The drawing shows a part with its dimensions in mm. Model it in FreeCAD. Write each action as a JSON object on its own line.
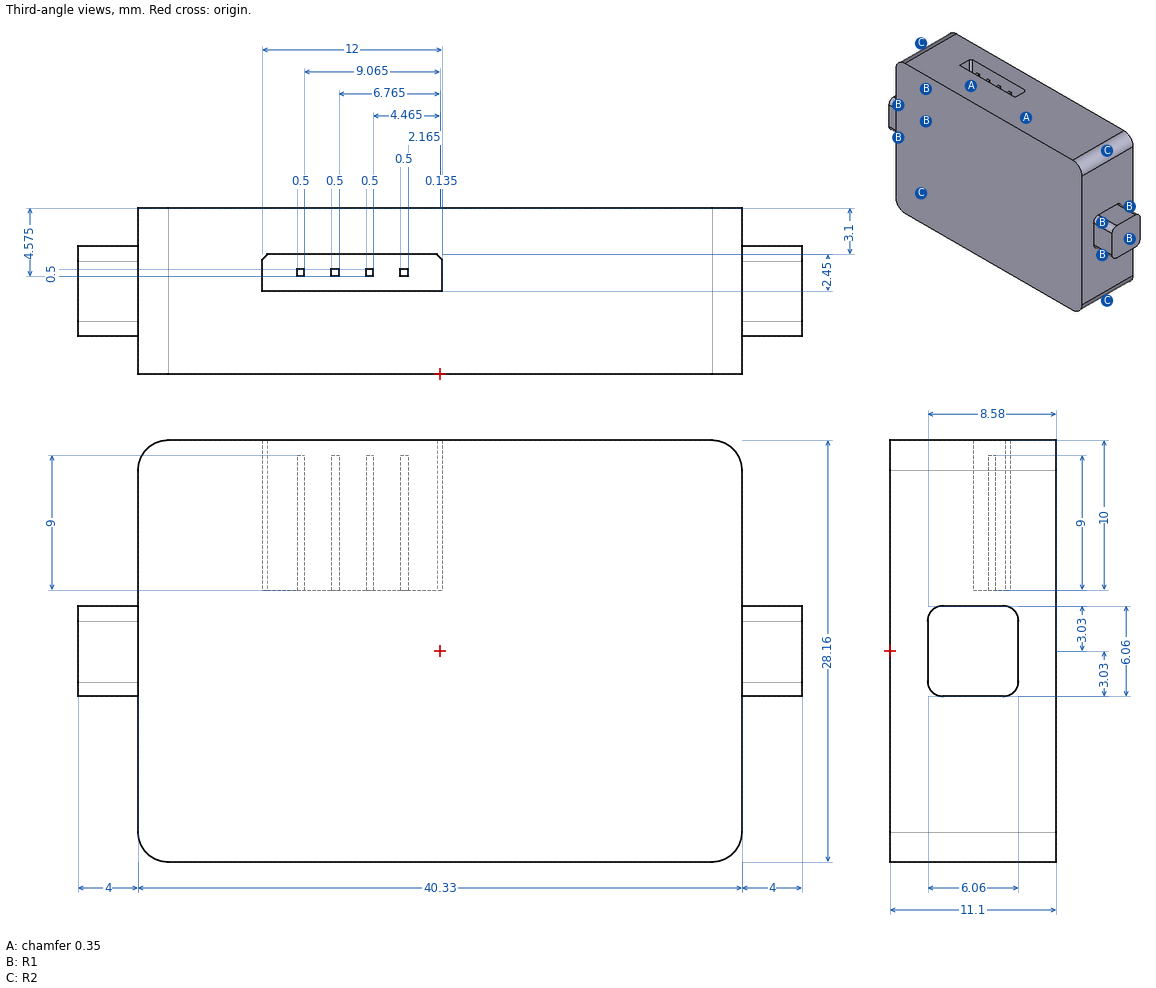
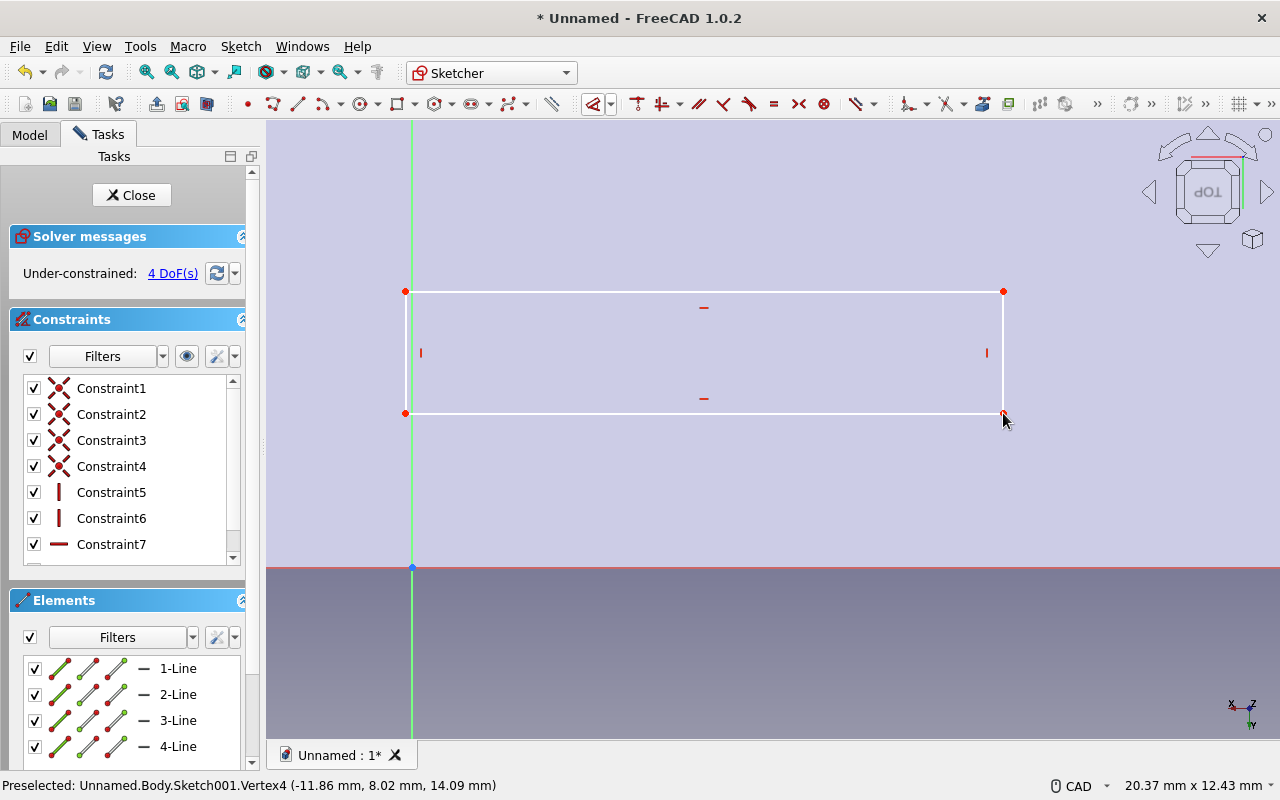
{"action": "key", "text": "d"}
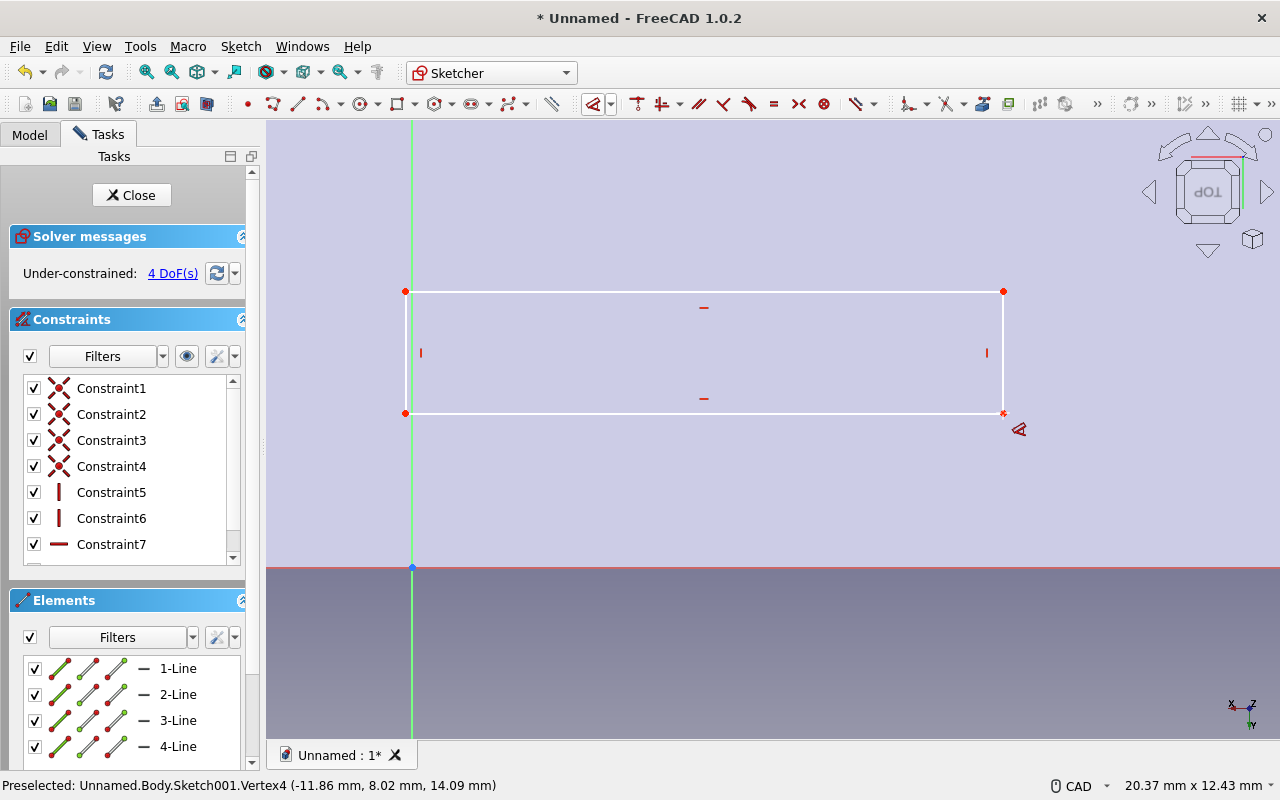
{"action": "left_click", "coordinate": [585, 414]}
{"action": "left_click", "coordinate": [704, 380]}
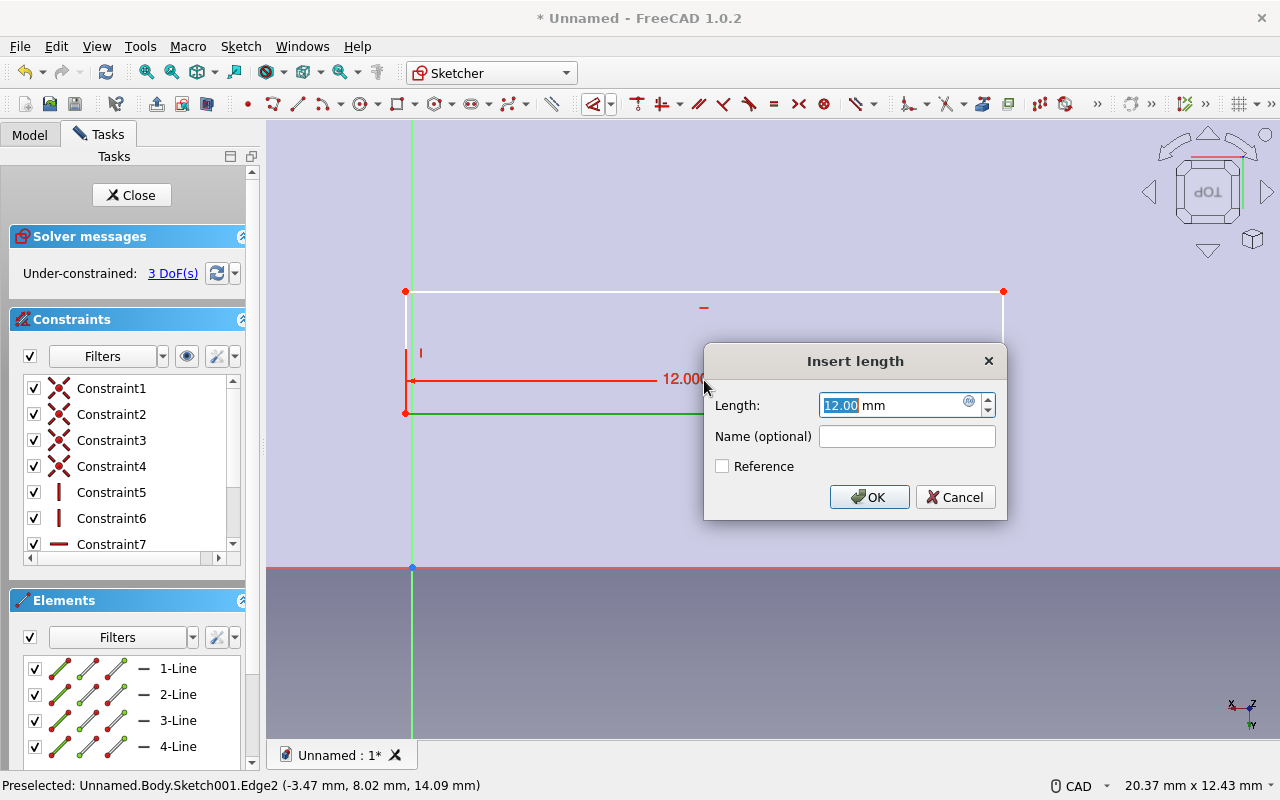
{"action": "type", "text": "12"}
{"action": "key", "text": "Return"}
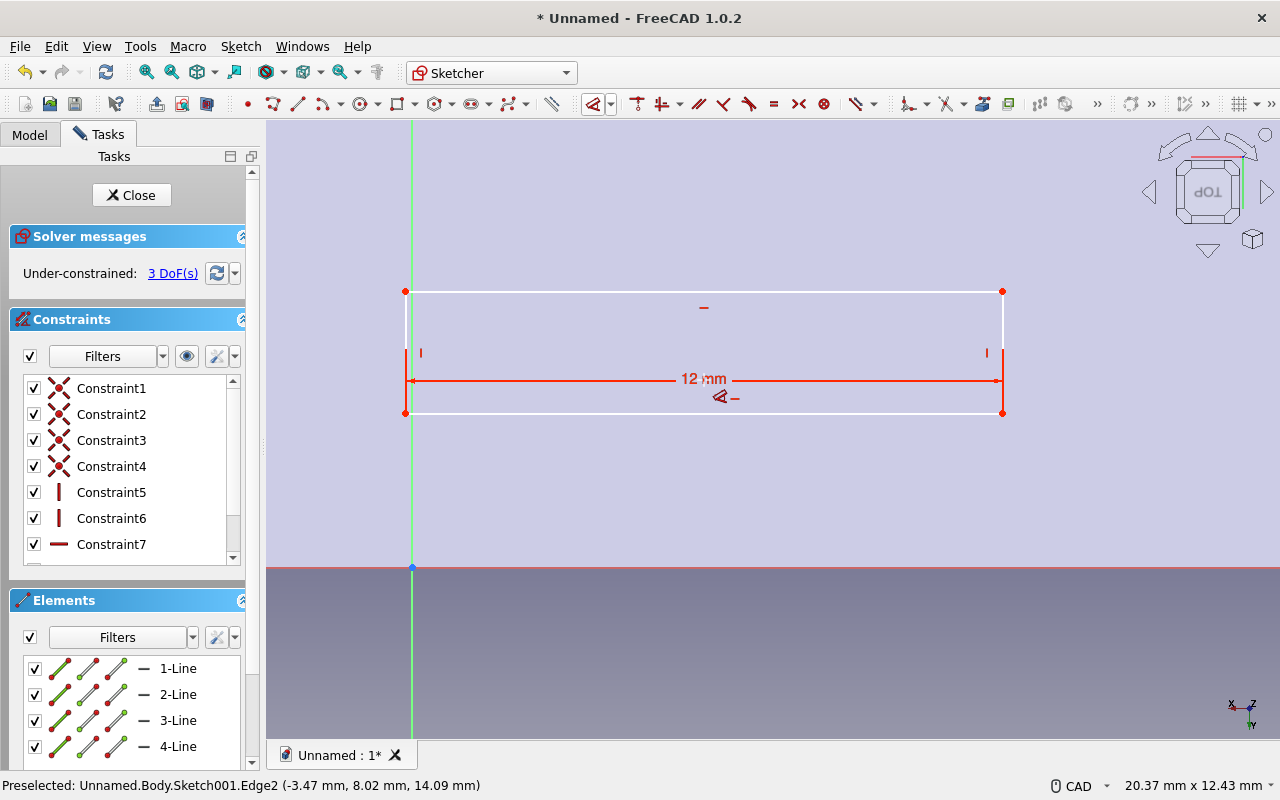
{"action": "scroll", "coordinate": [406, 328], "scroll_direction": "up", "scroll_amount": 4}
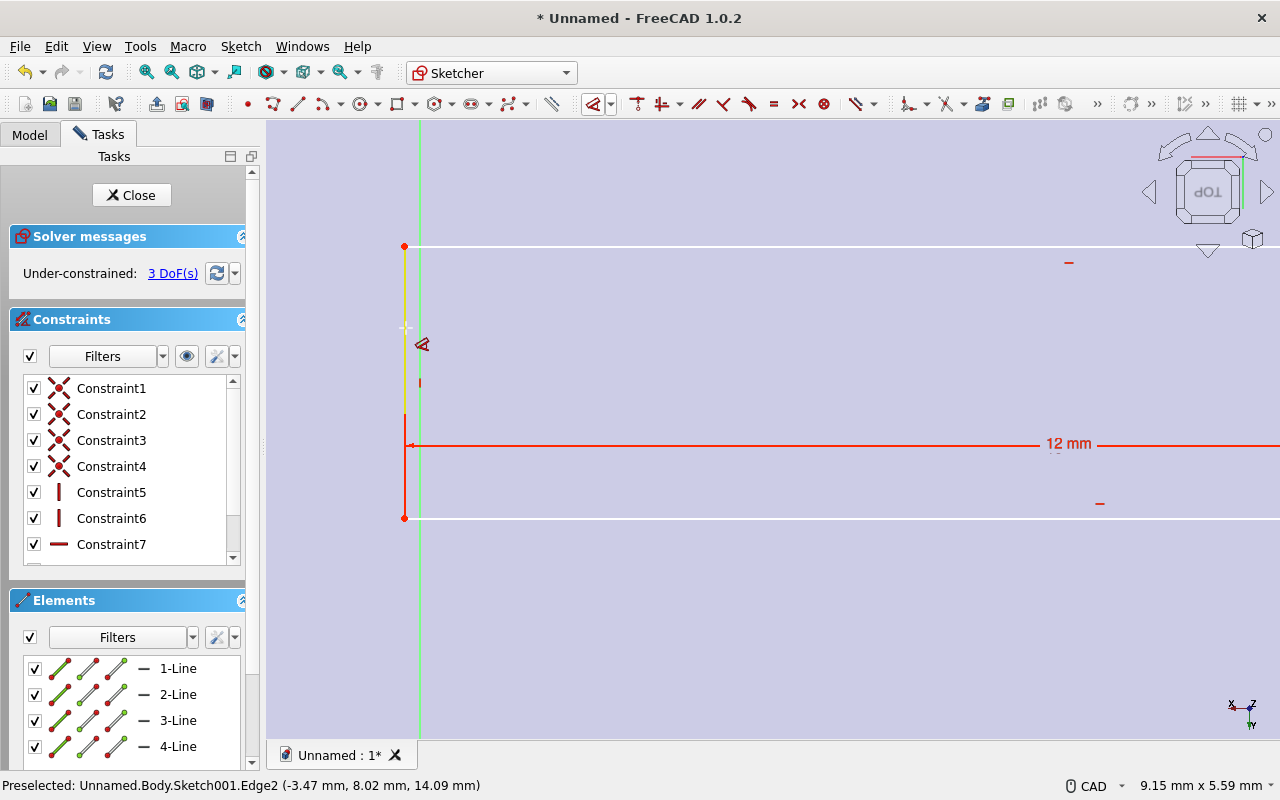
{"action": "left_click", "coordinate": [405, 328]}
{"action": "left_click", "coordinate": [371, 383]}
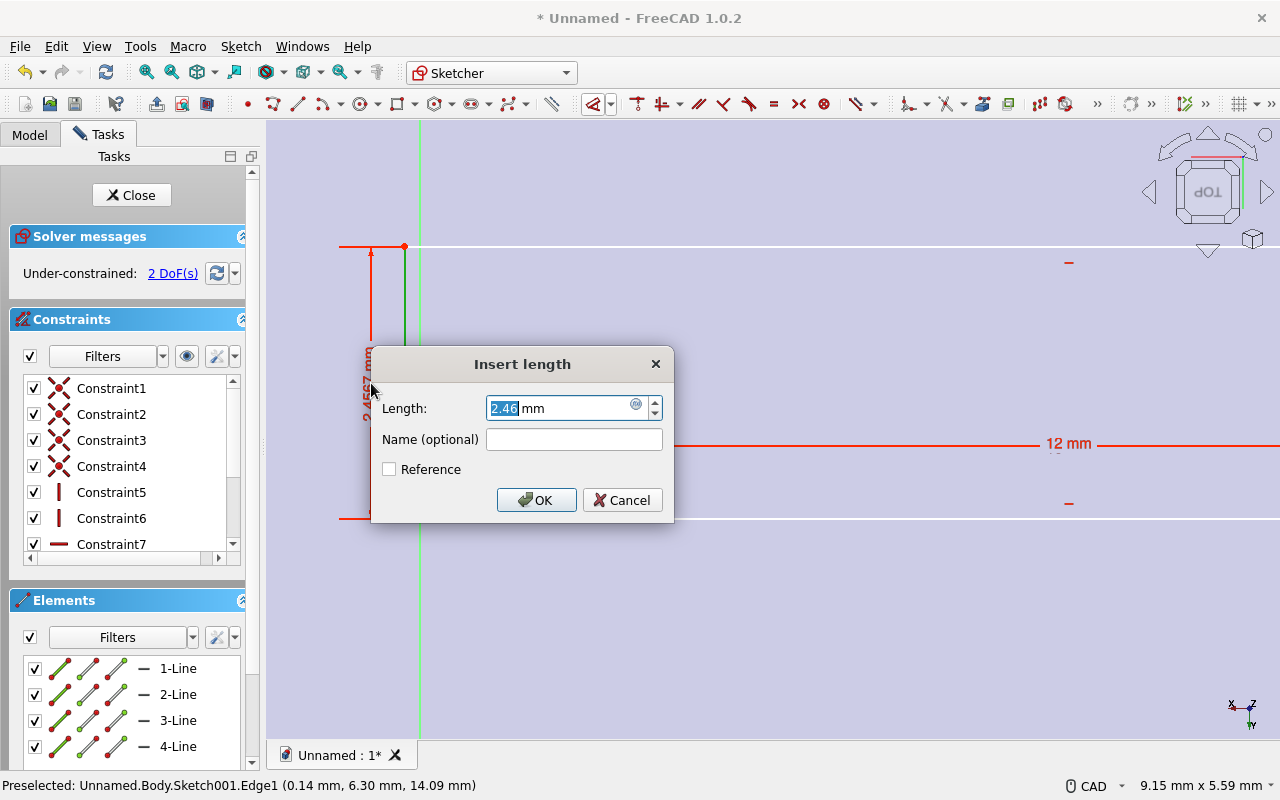
{"action": "type", "text": "2.45"}
{"action": "key", "text": "Return"}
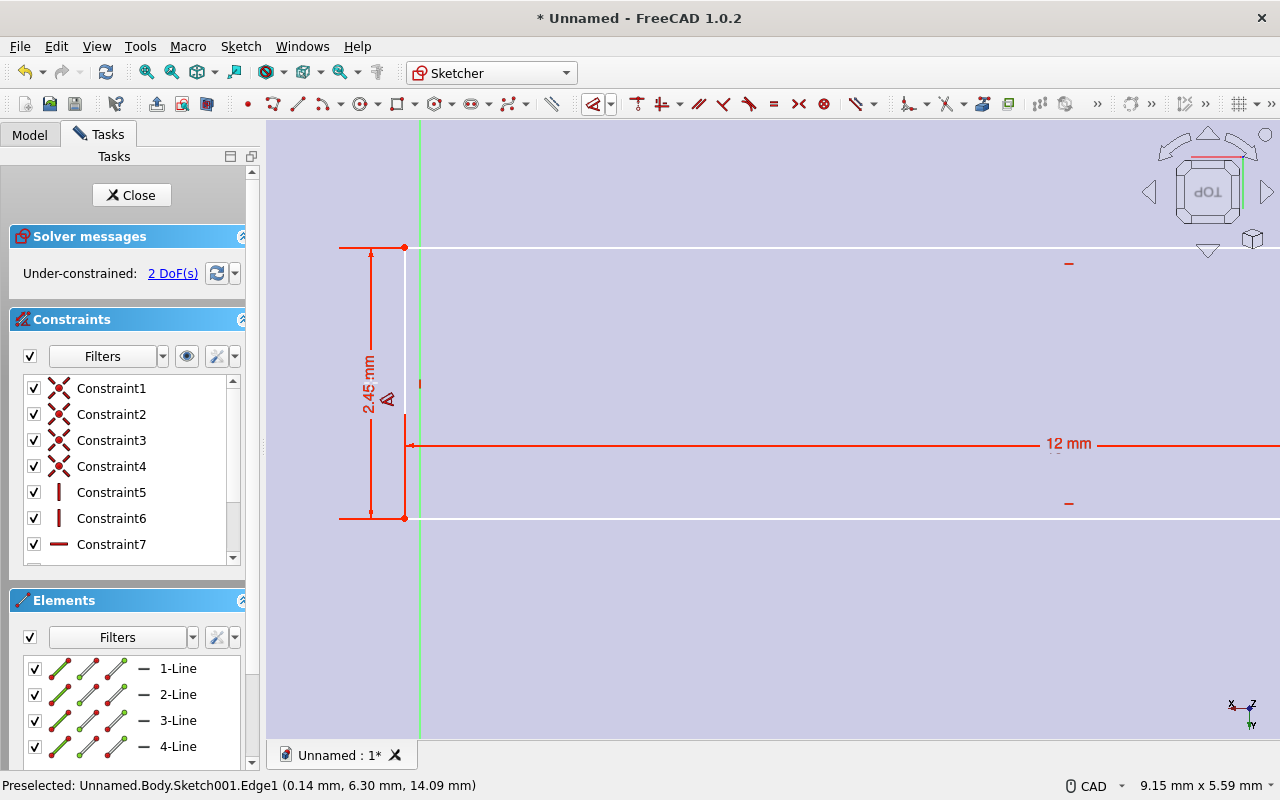
{"action": "left_click", "coordinate": [405, 519]}
{"action": "left_click", "coordinate": [371, 615]}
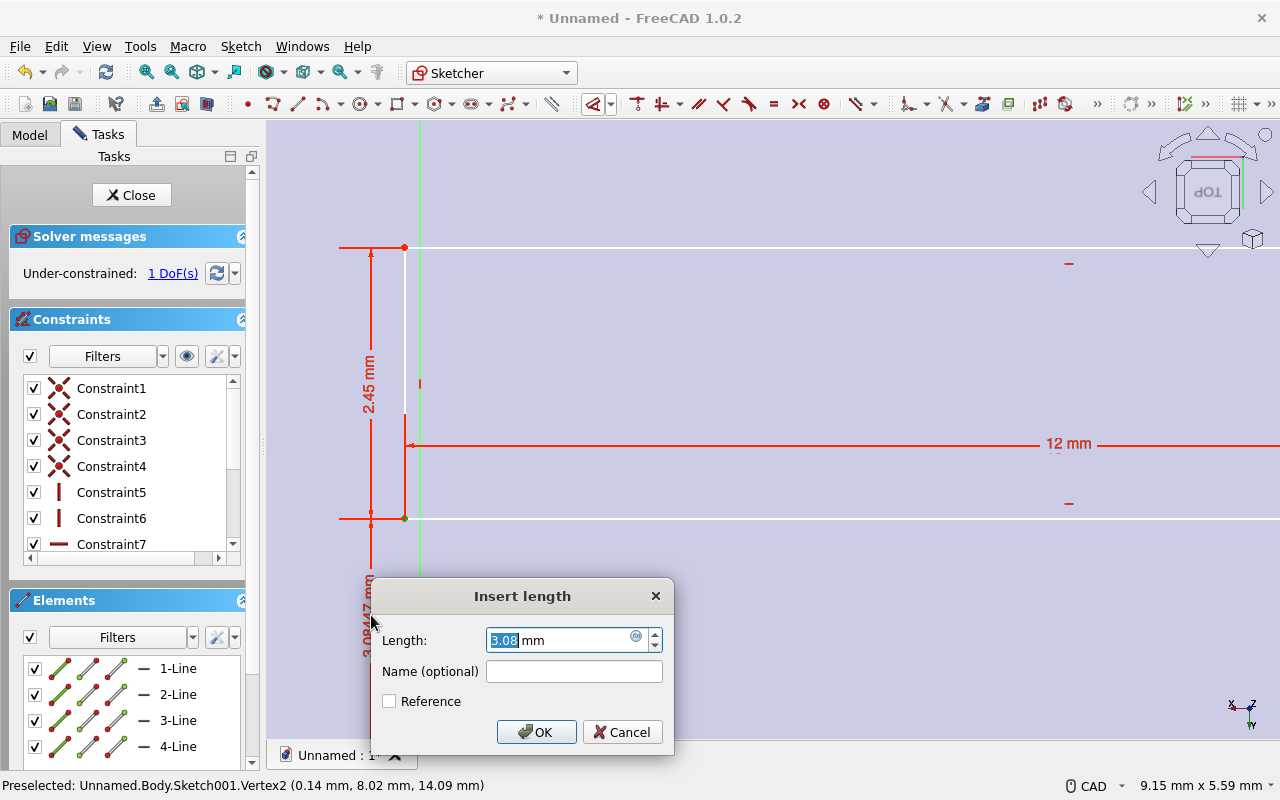
{"action": "type", "text": "3.1"}
{"action": "key", "text": "Return"}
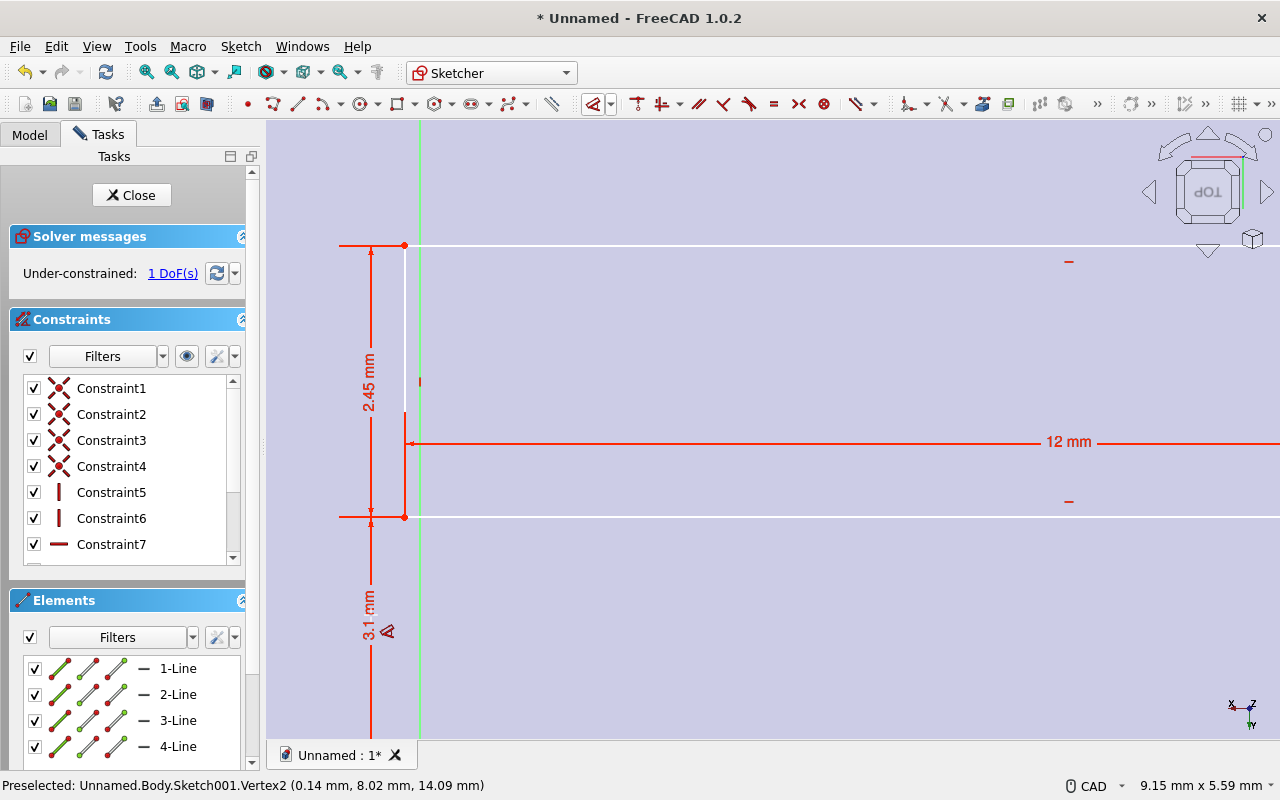
{"action": "scroll", "coordinate": [405, 246], "scroll_direction": "up", "scroll_amount": 5}